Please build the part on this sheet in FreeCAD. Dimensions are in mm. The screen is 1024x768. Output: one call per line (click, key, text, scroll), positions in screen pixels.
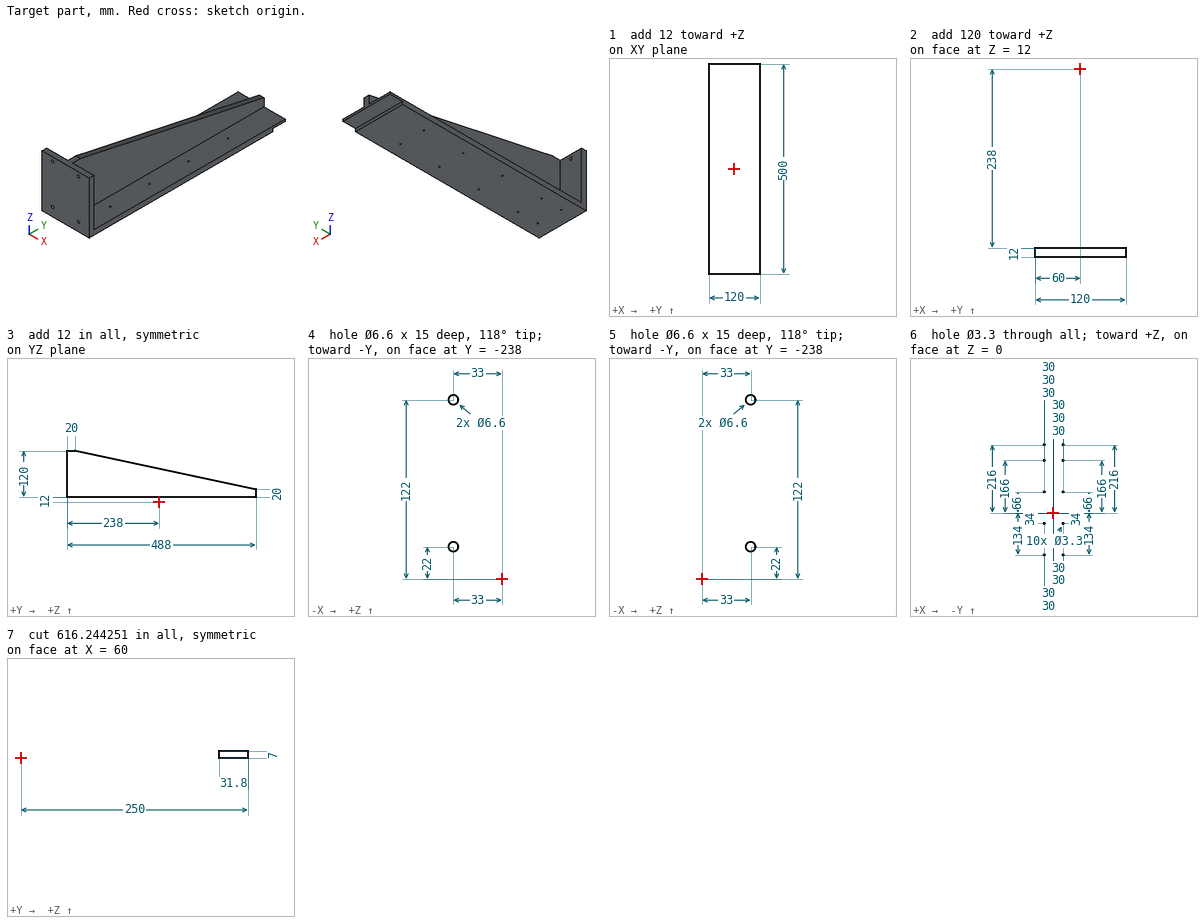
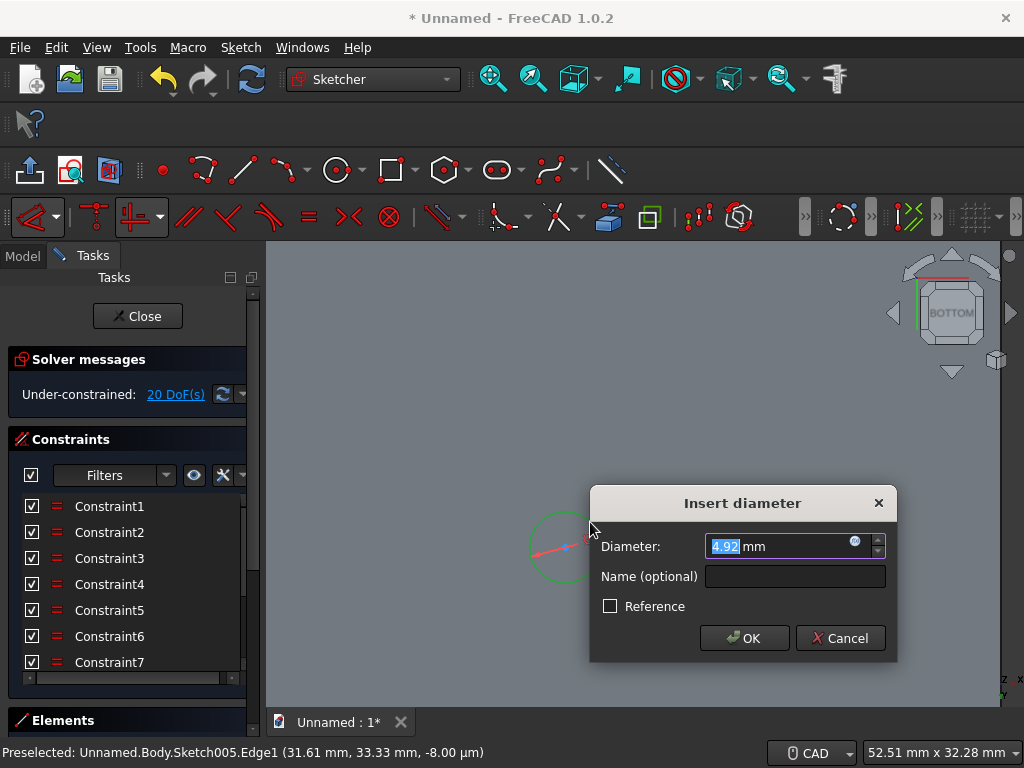
text(3.3)
key(Return)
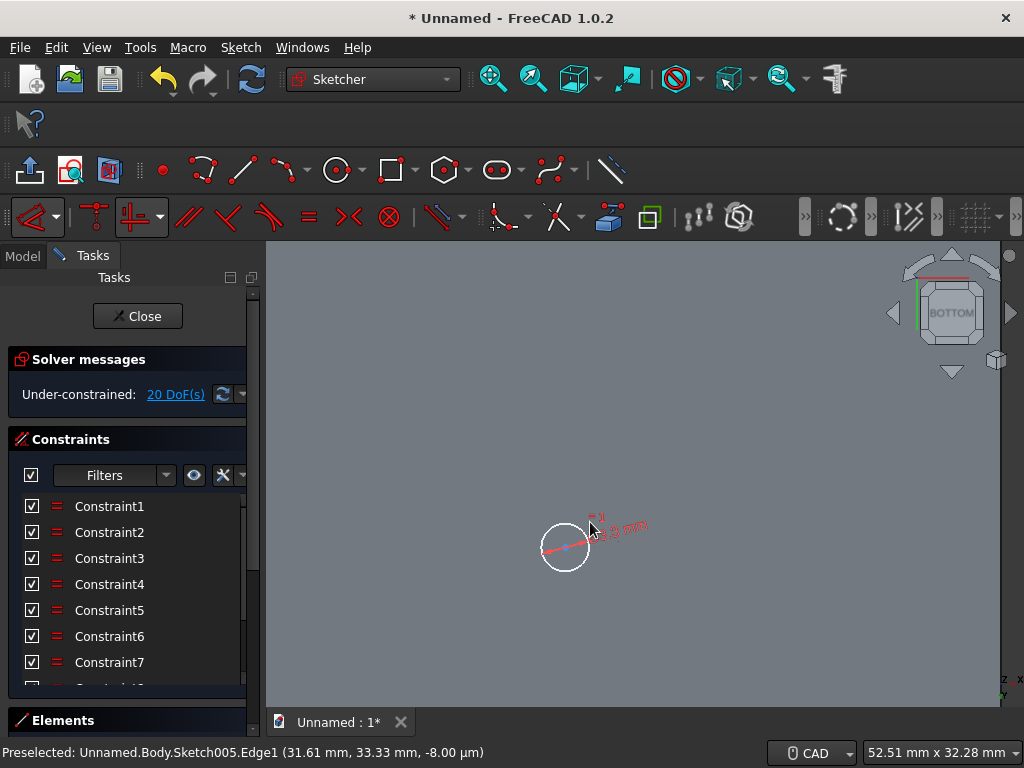
scroll(605, 540, down, 14)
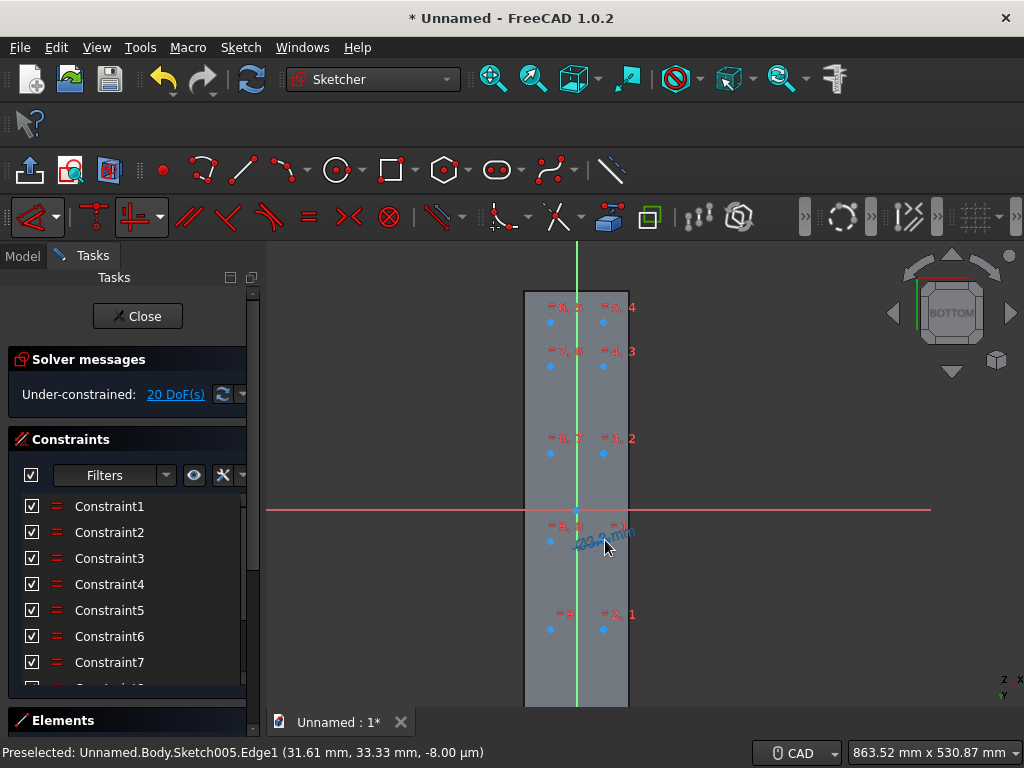
scroll(603, 541, up, 3)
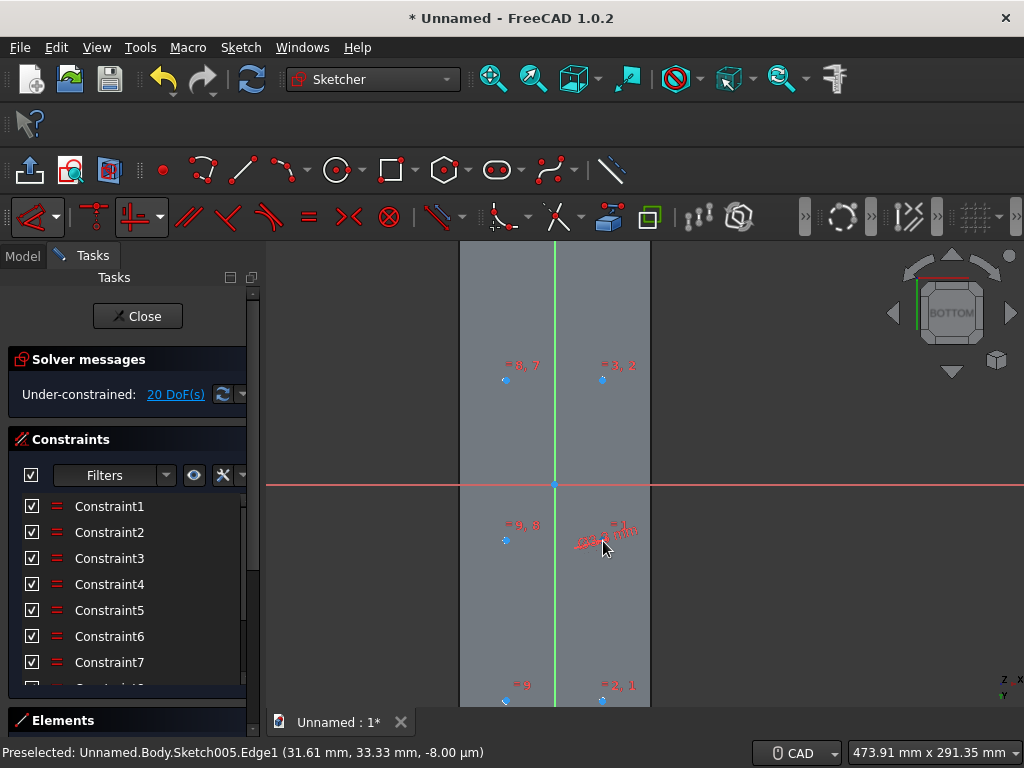
click(603, 541)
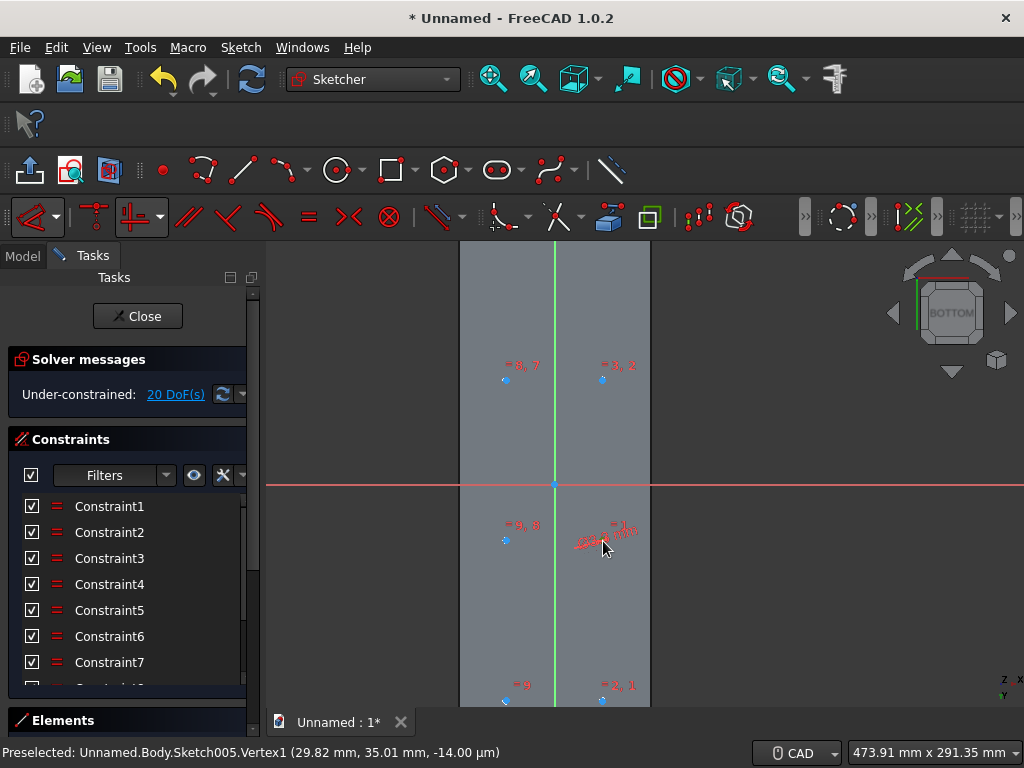
key(l)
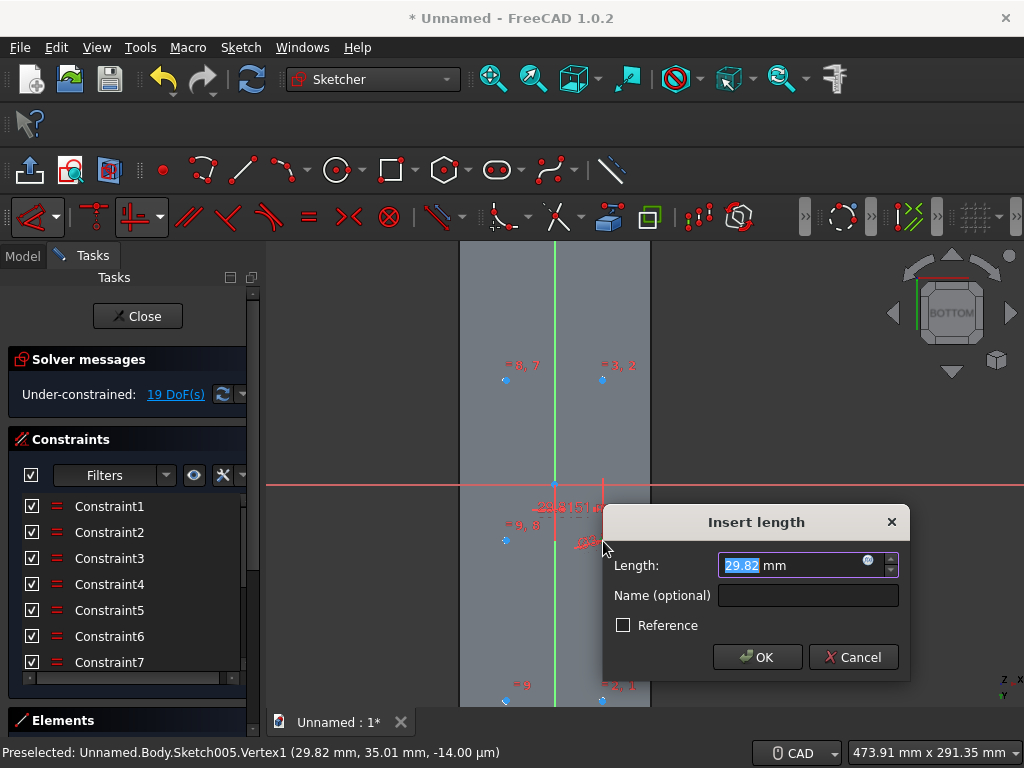
text(30)
key(Return)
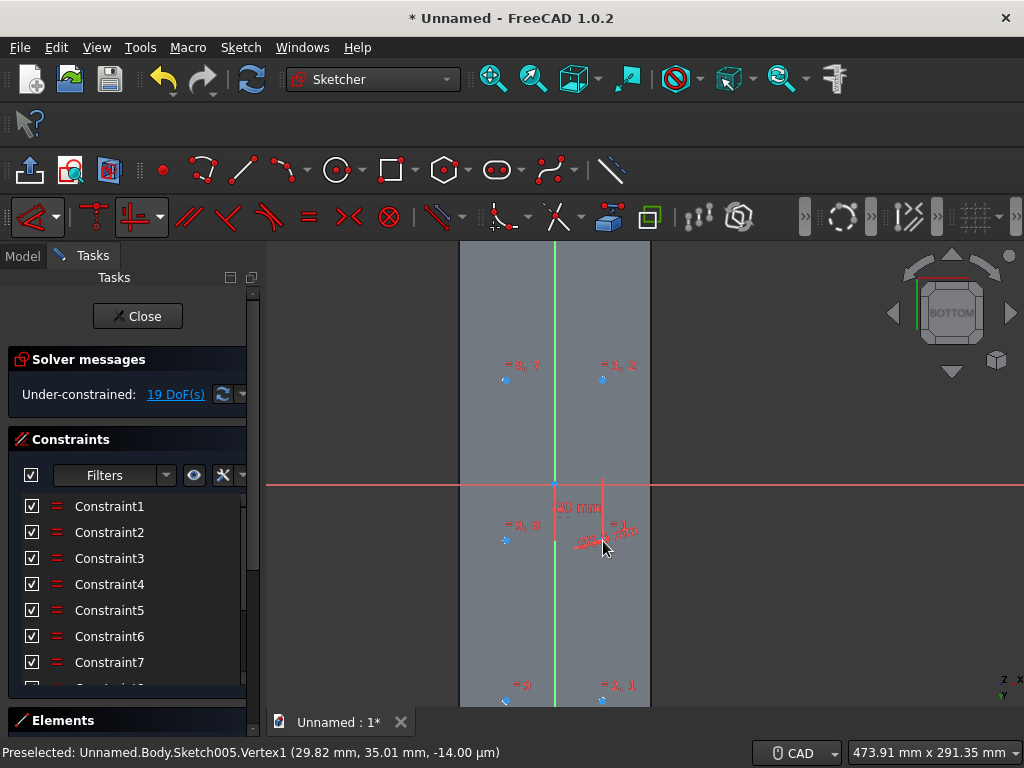
click(603, 541)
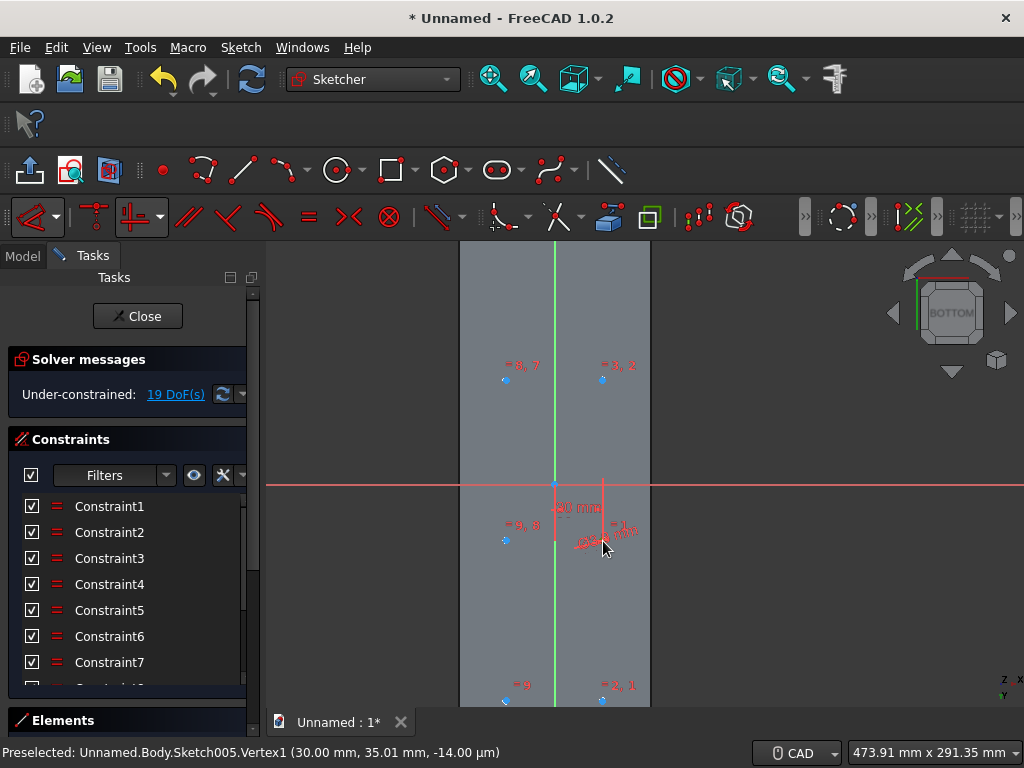
click(58, 218)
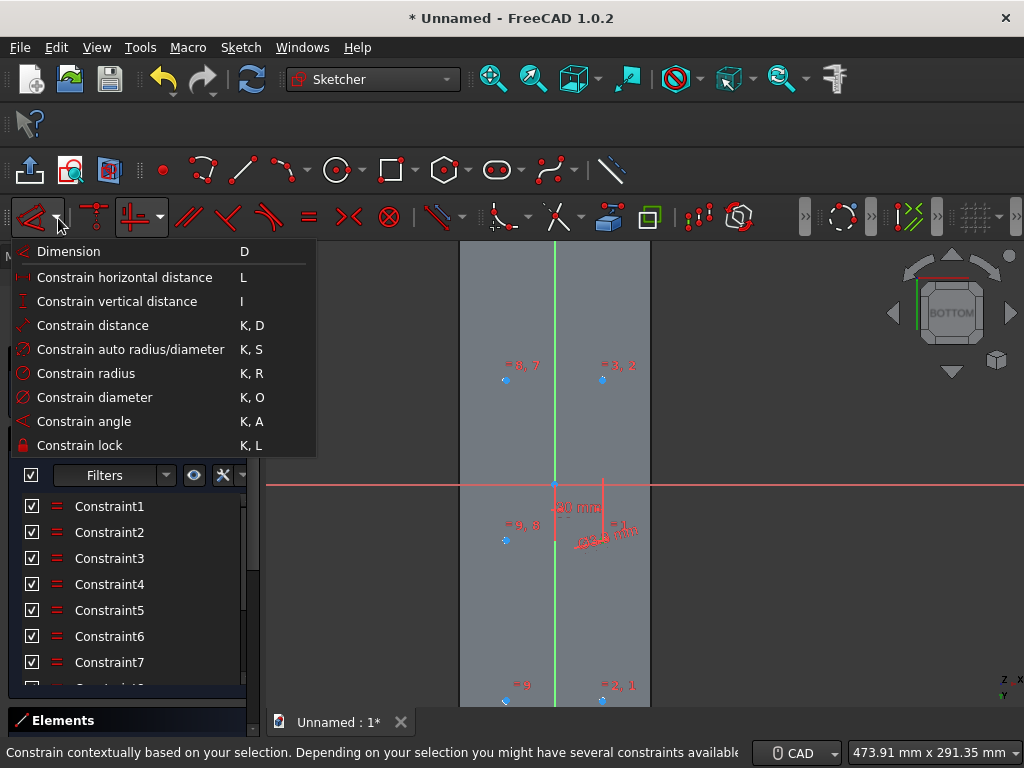
click(164, 301)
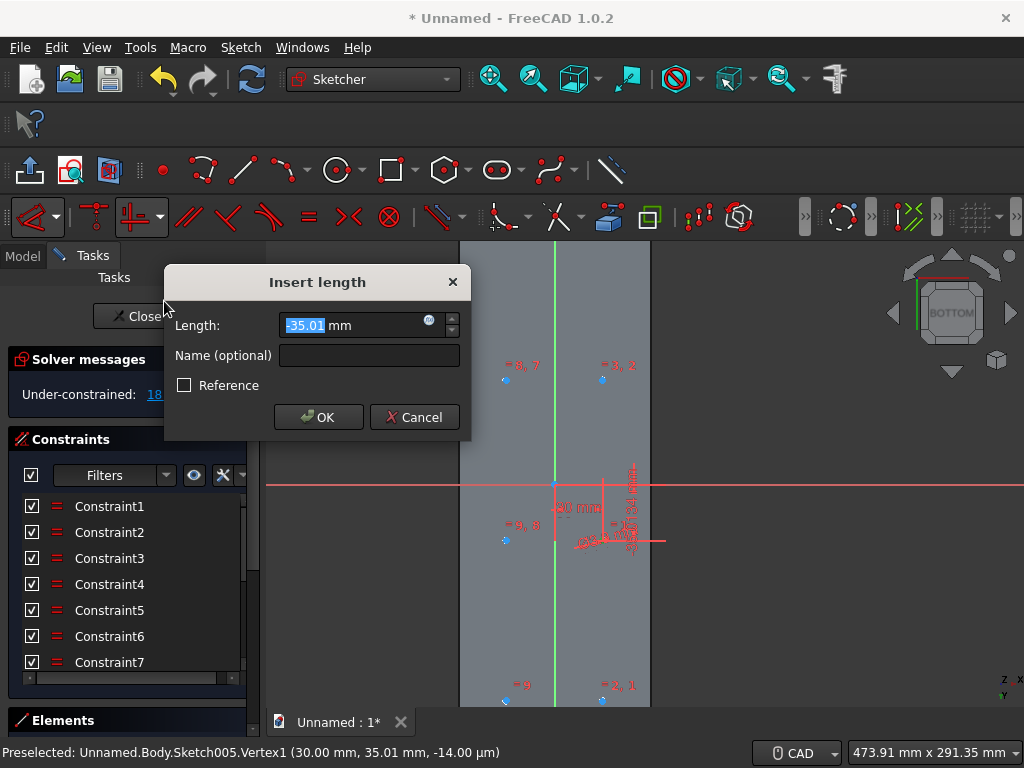
text(-34)
key(Return)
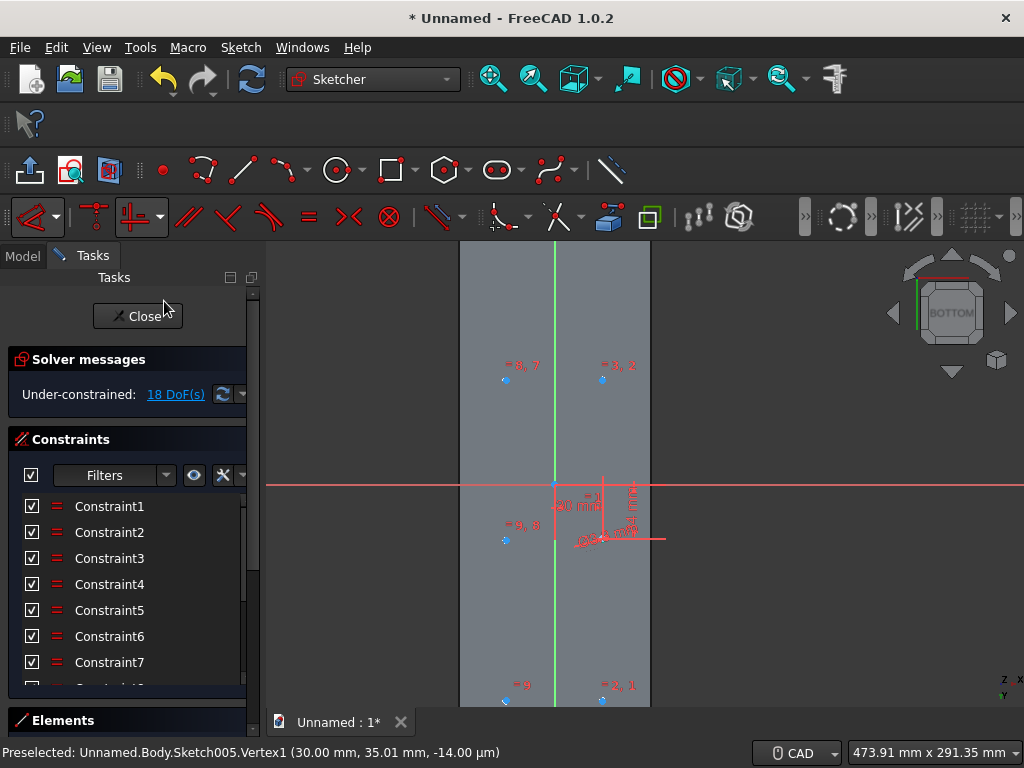
scroll(603, 541, down, 3)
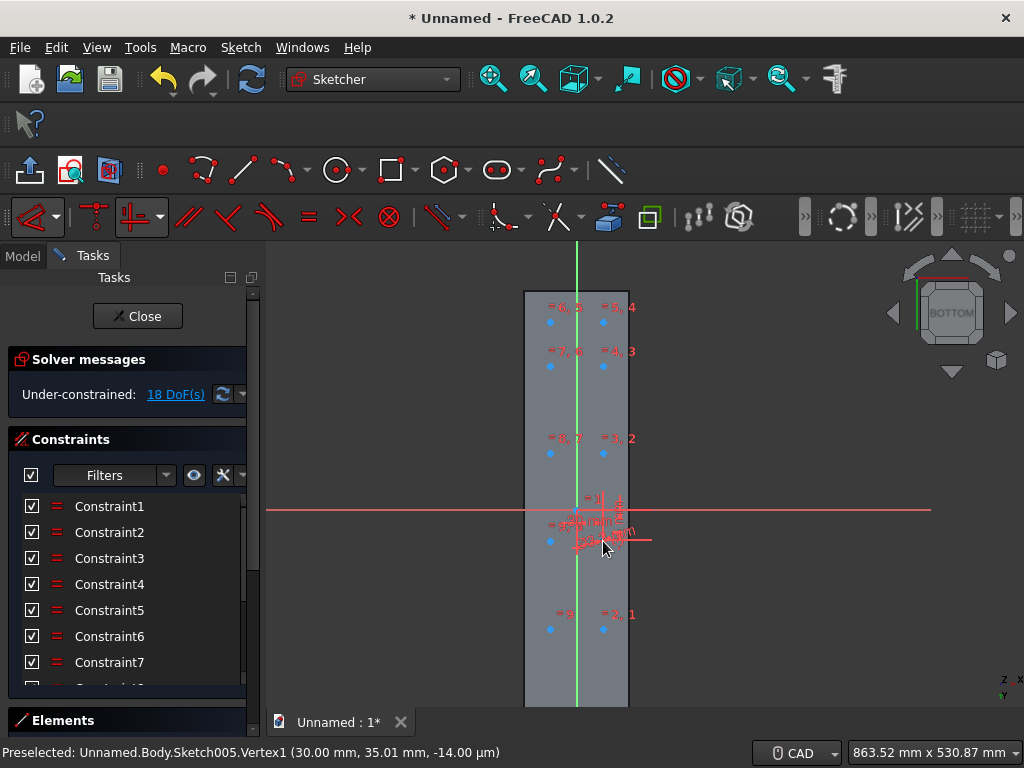
scroll(603, 629, up, 3)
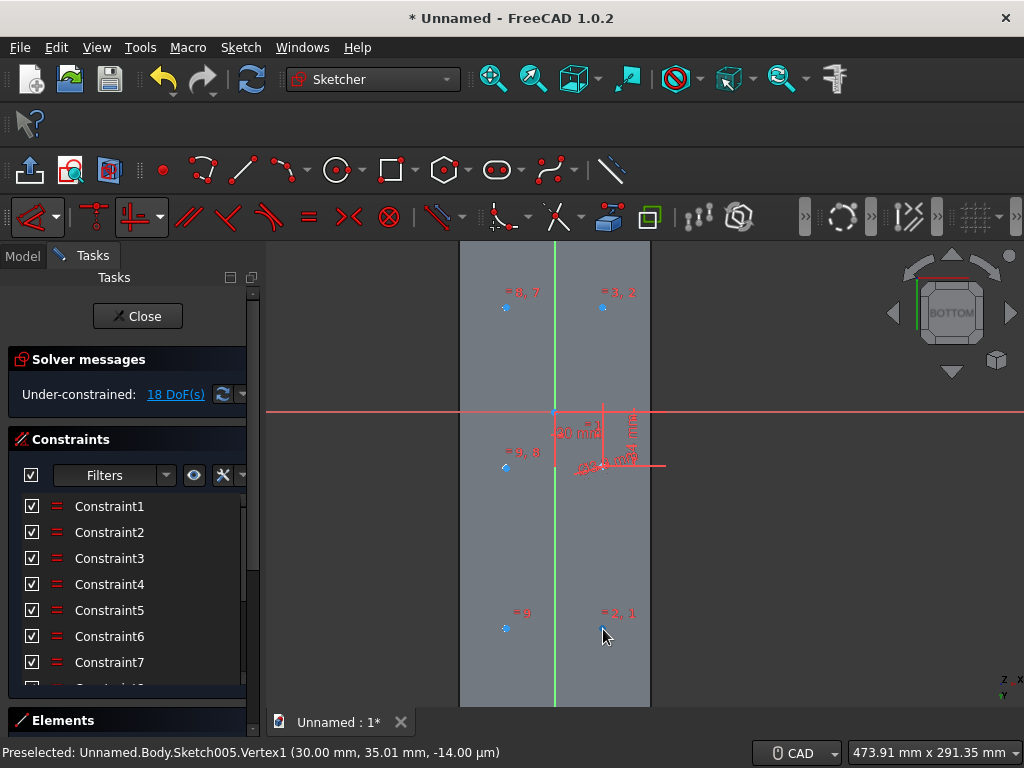
click(603, 629)